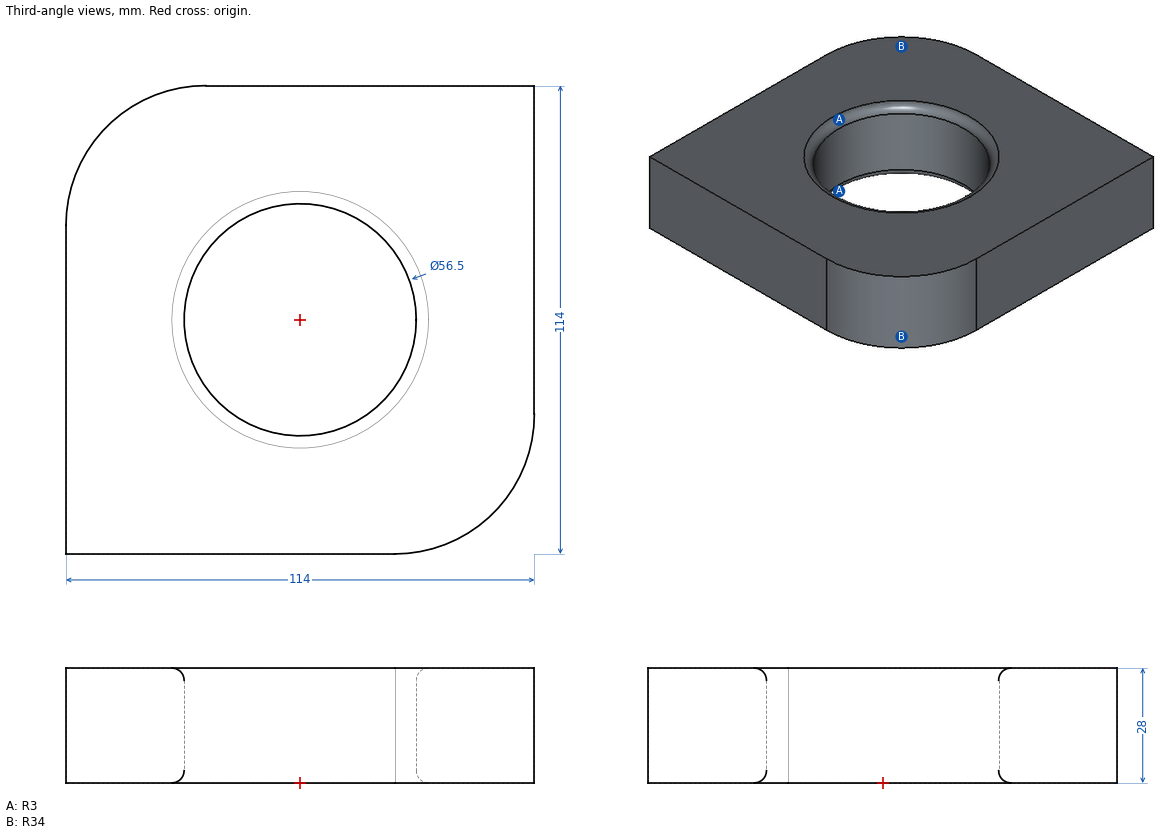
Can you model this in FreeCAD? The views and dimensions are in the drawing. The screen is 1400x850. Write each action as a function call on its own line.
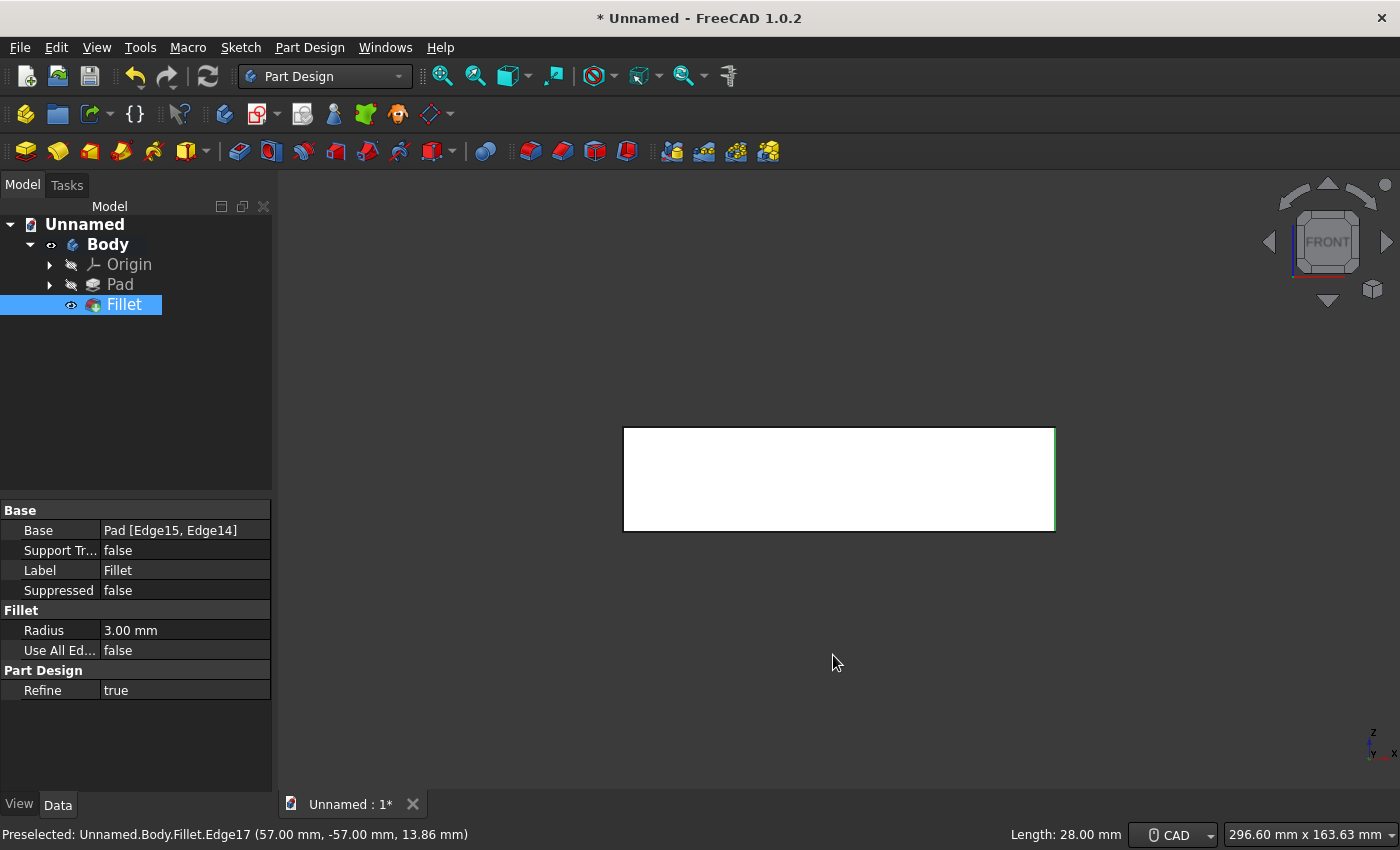
key(v)
key(f)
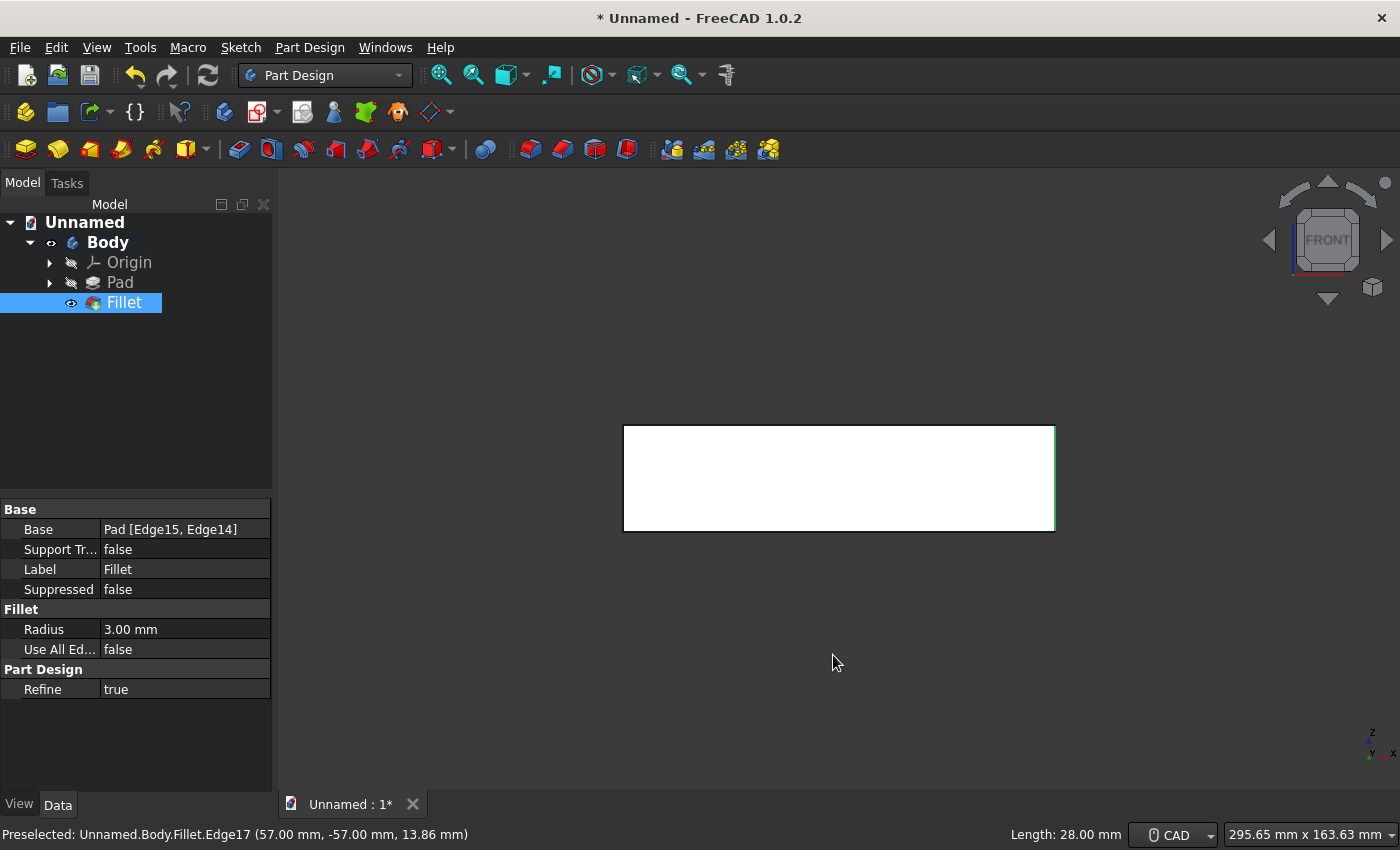
key(3)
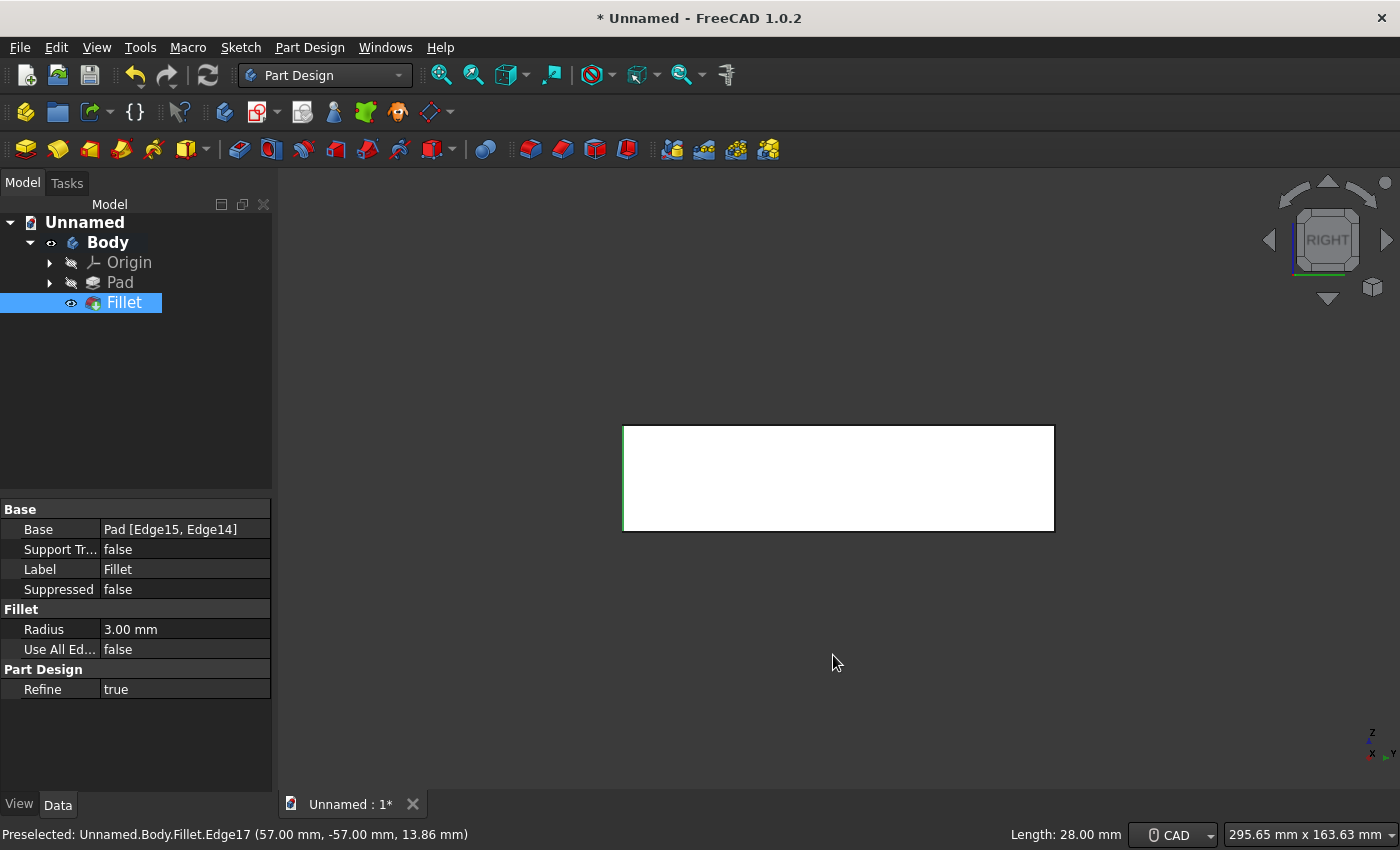
key(v)
key(f)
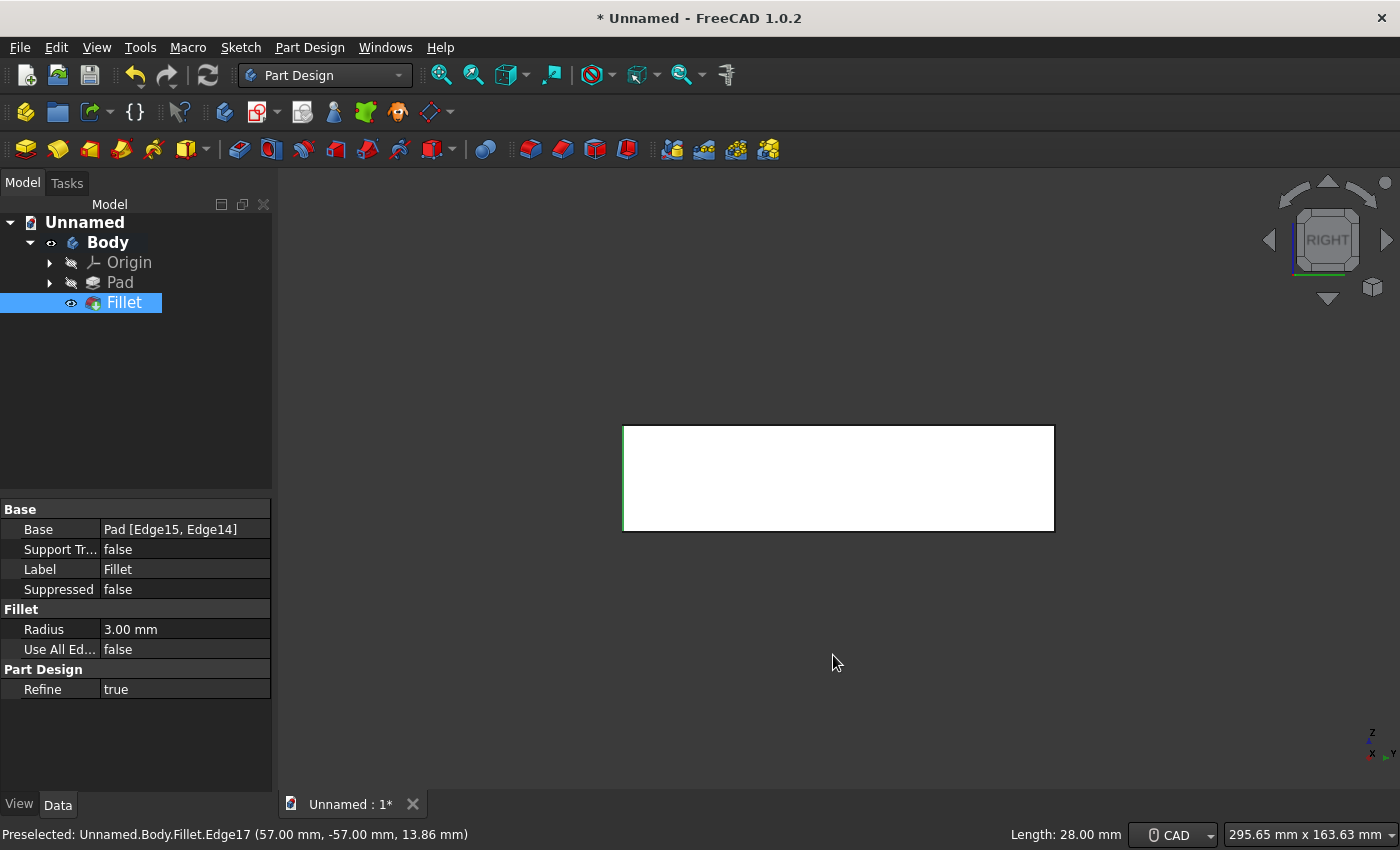
key(5)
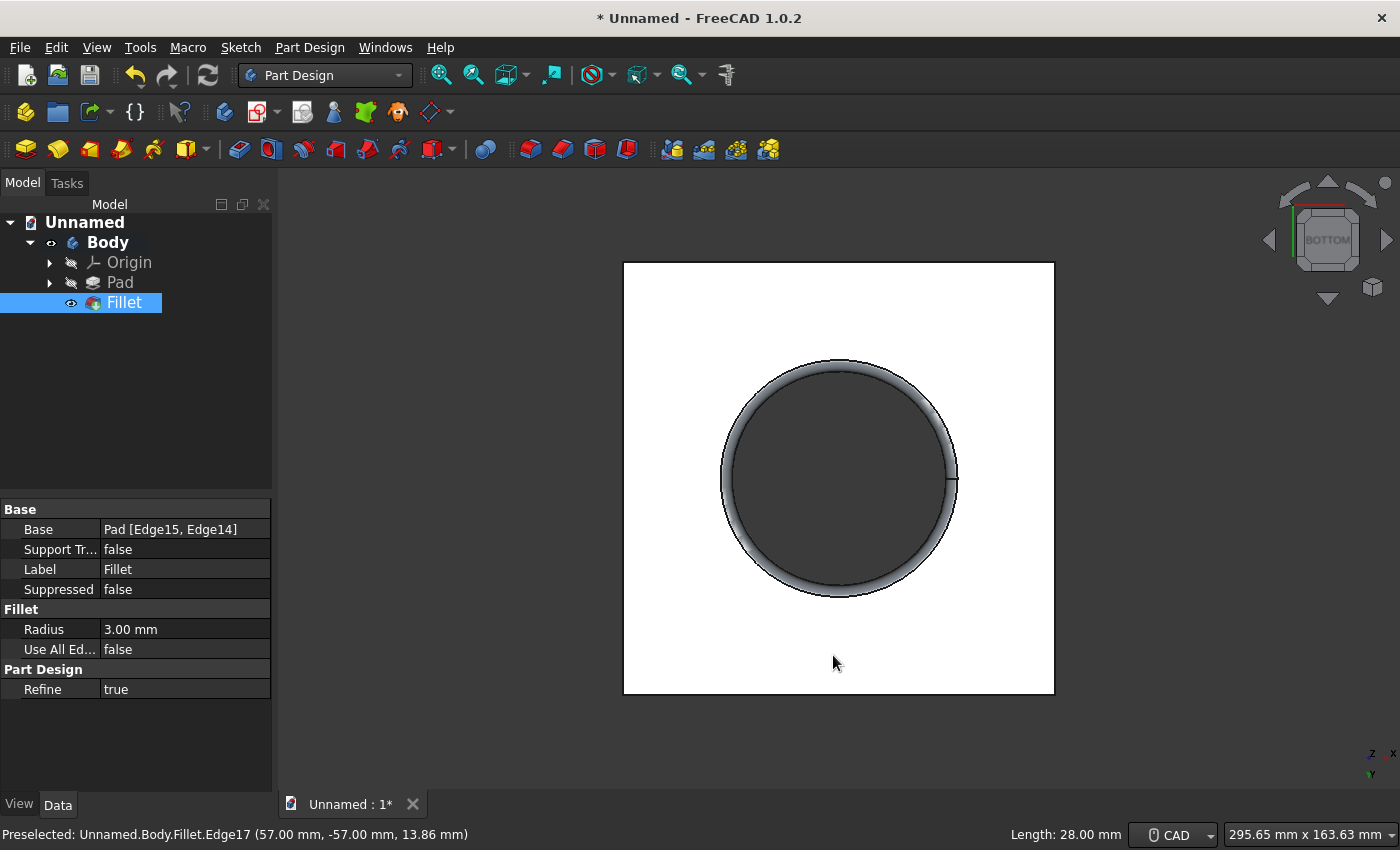
key(4)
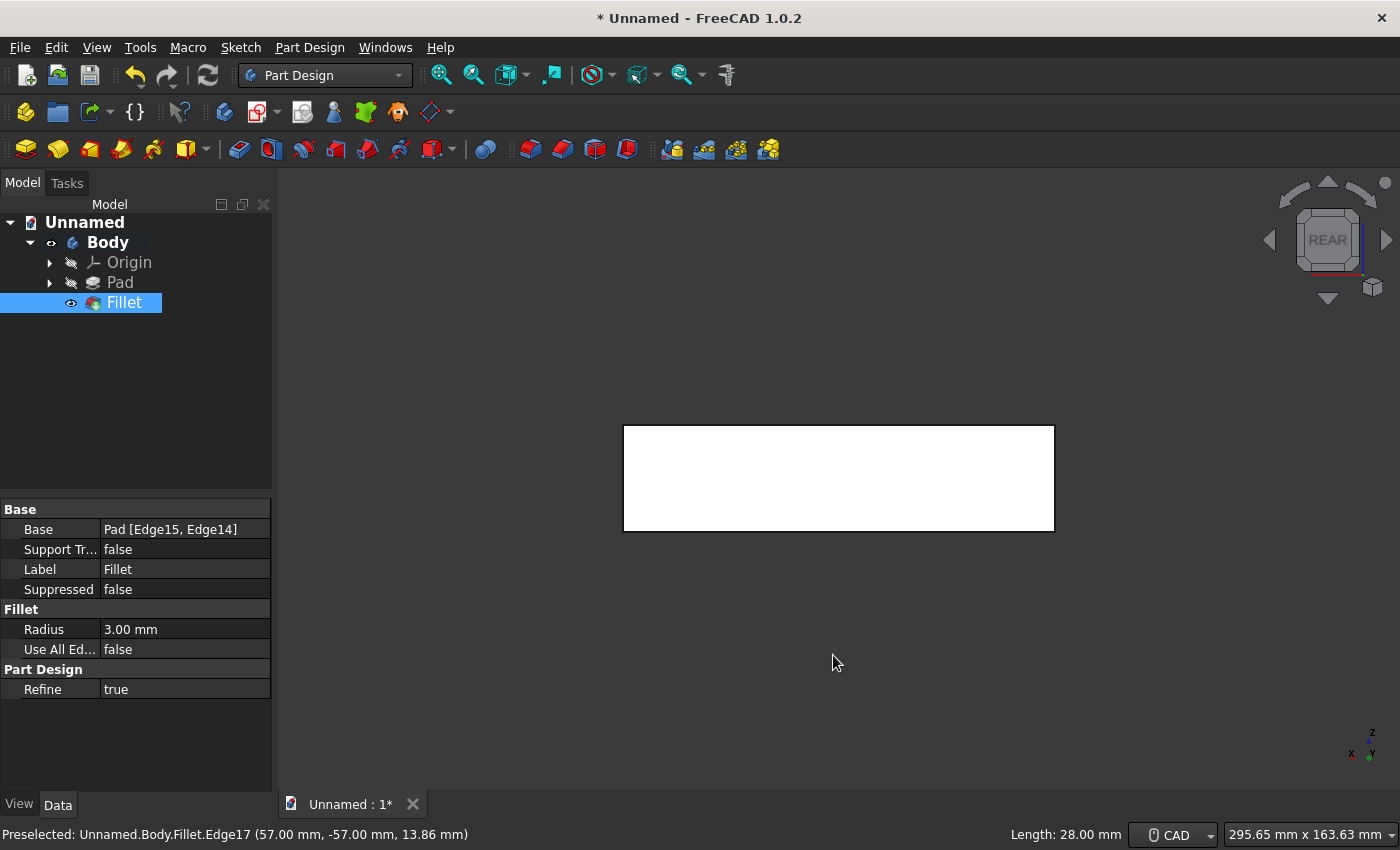
click(442, 76)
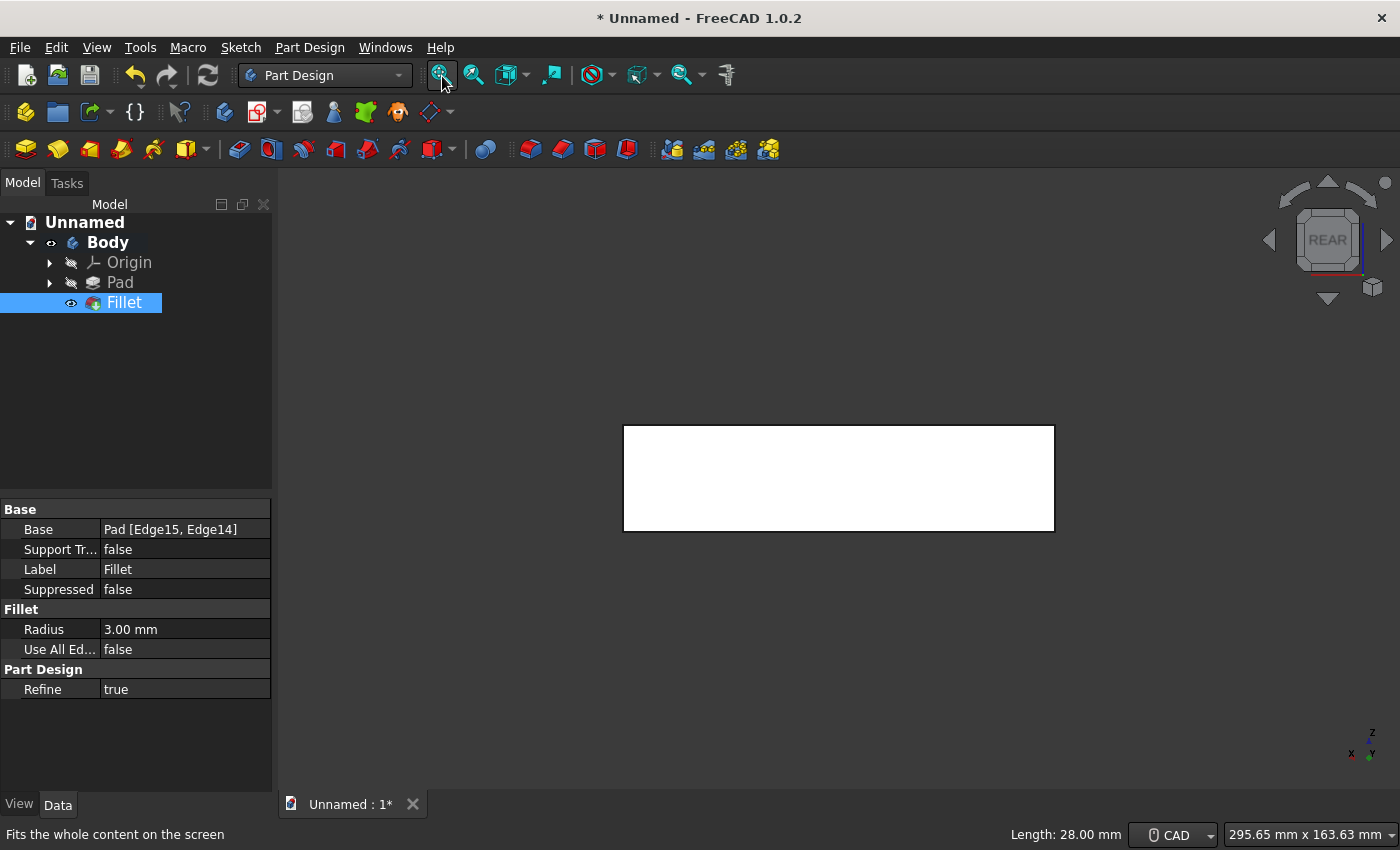
click(1055, 478, ctrl)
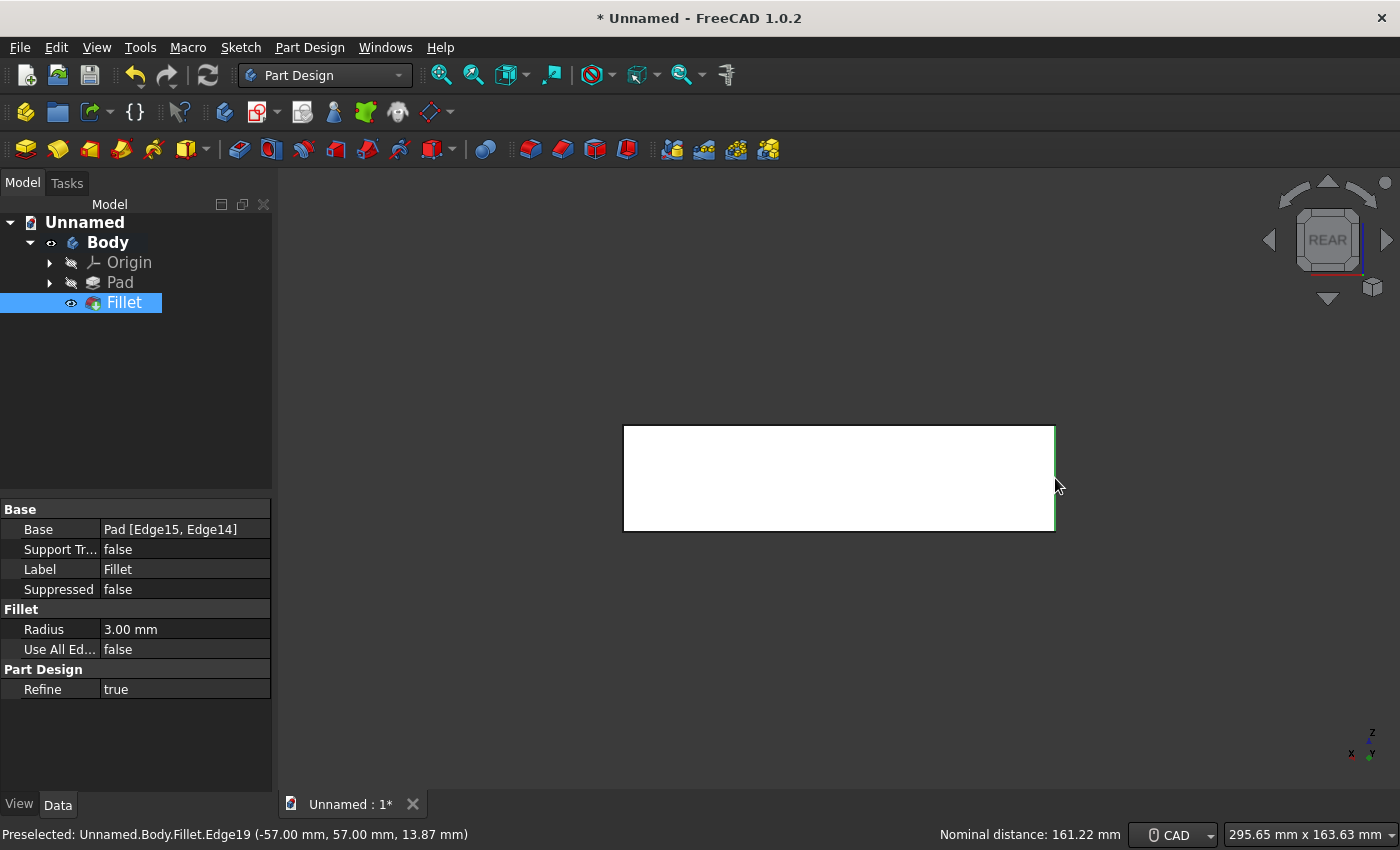
click(532, 150)